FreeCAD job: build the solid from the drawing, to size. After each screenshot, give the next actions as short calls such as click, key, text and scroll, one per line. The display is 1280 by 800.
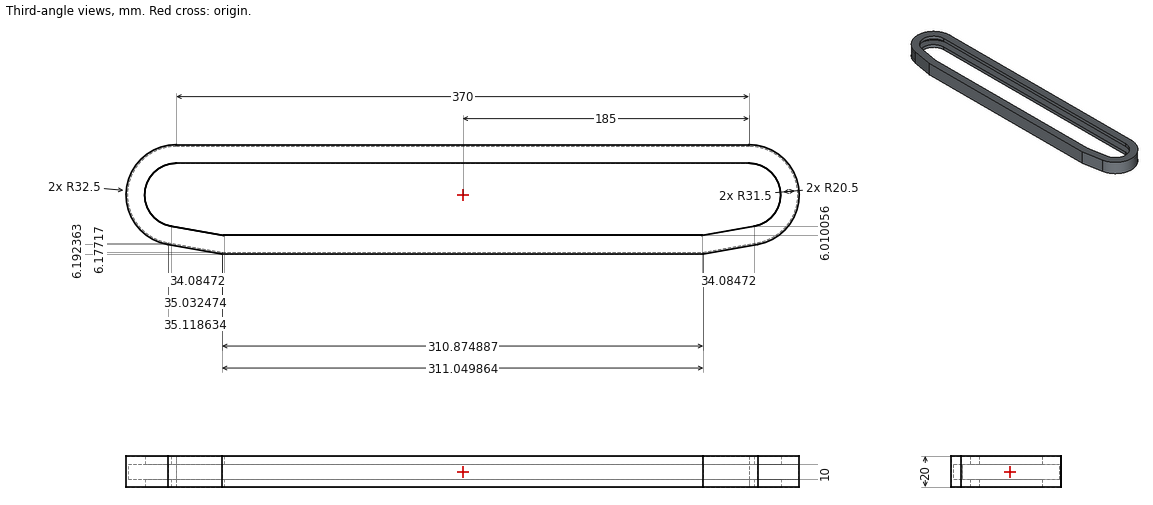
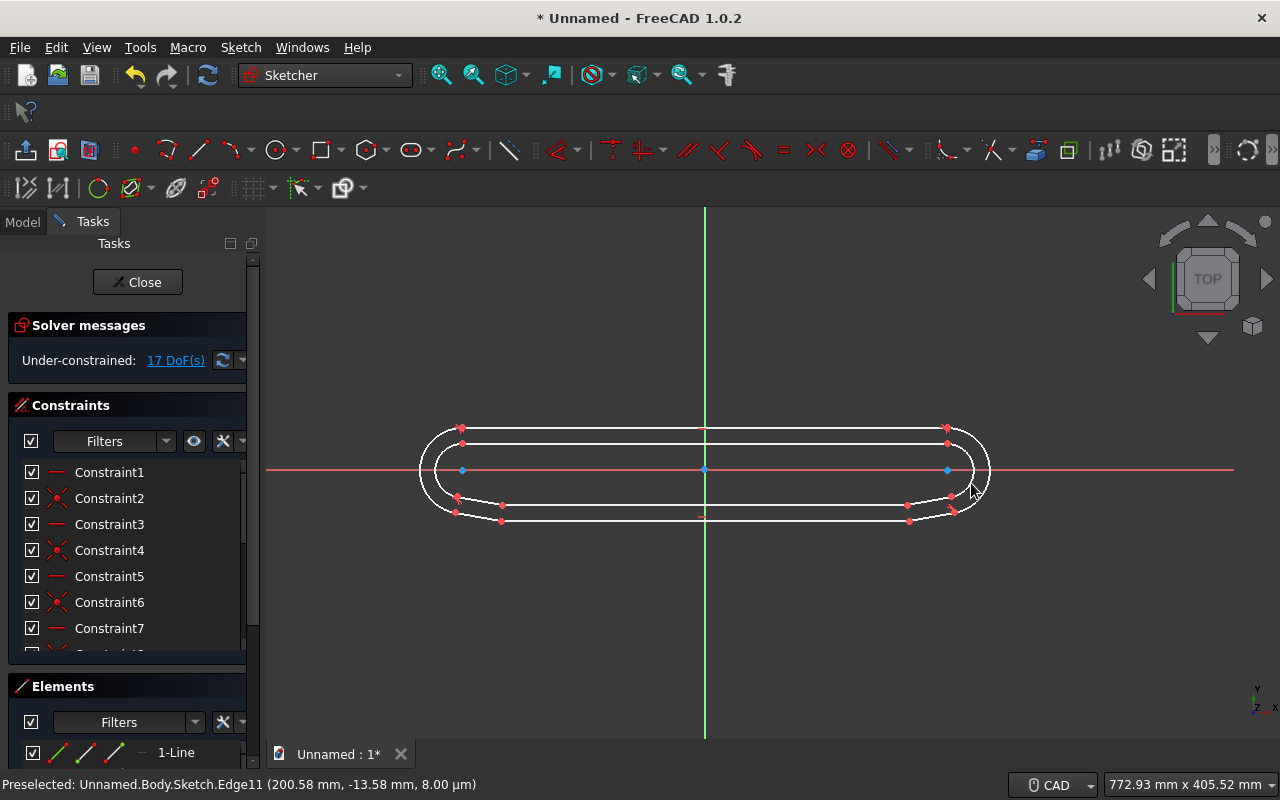
click(489, 503)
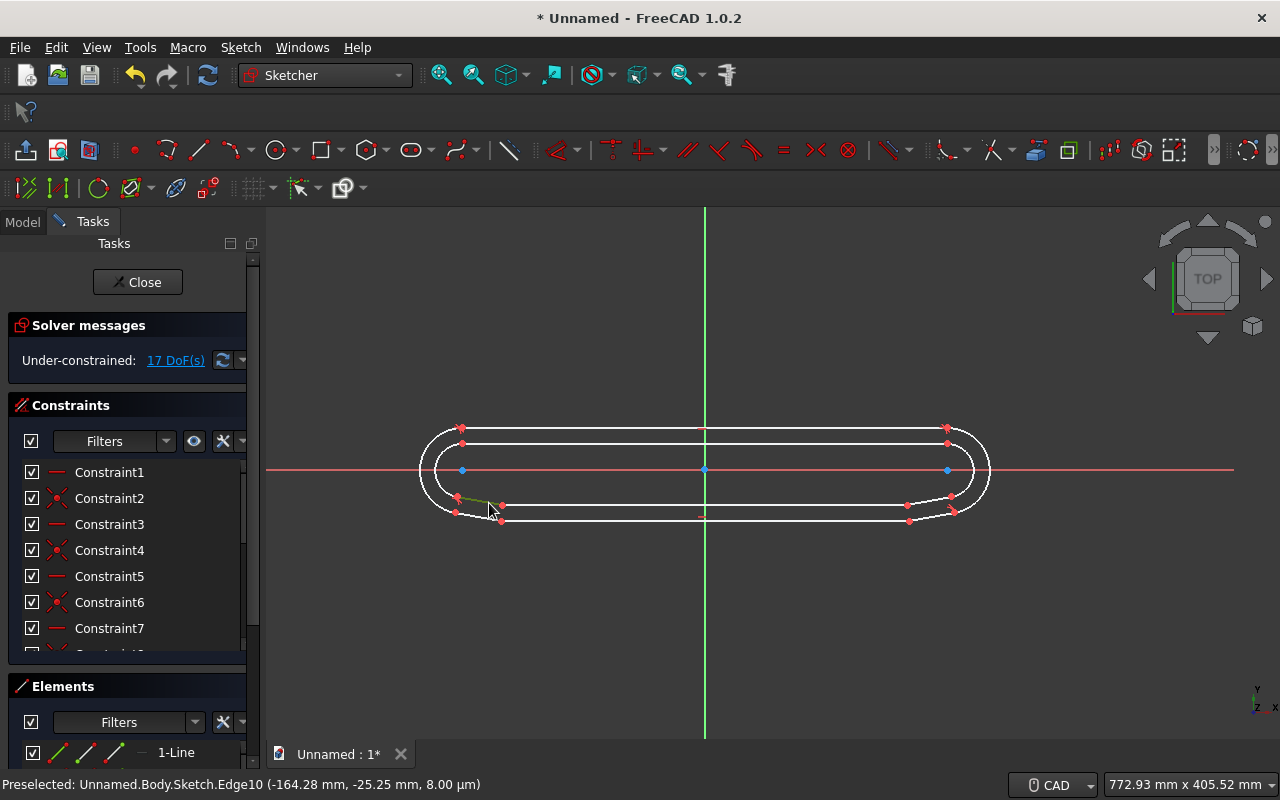
click(441, 454)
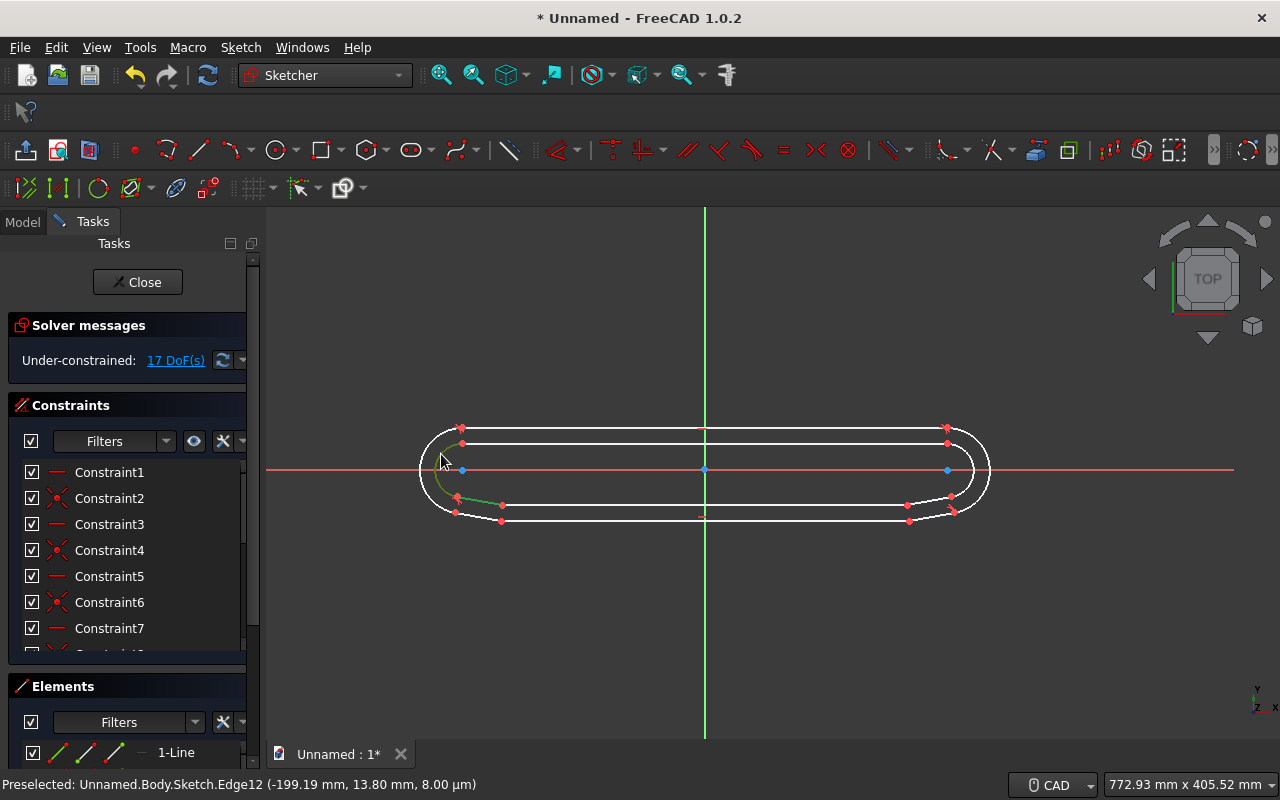
key(t)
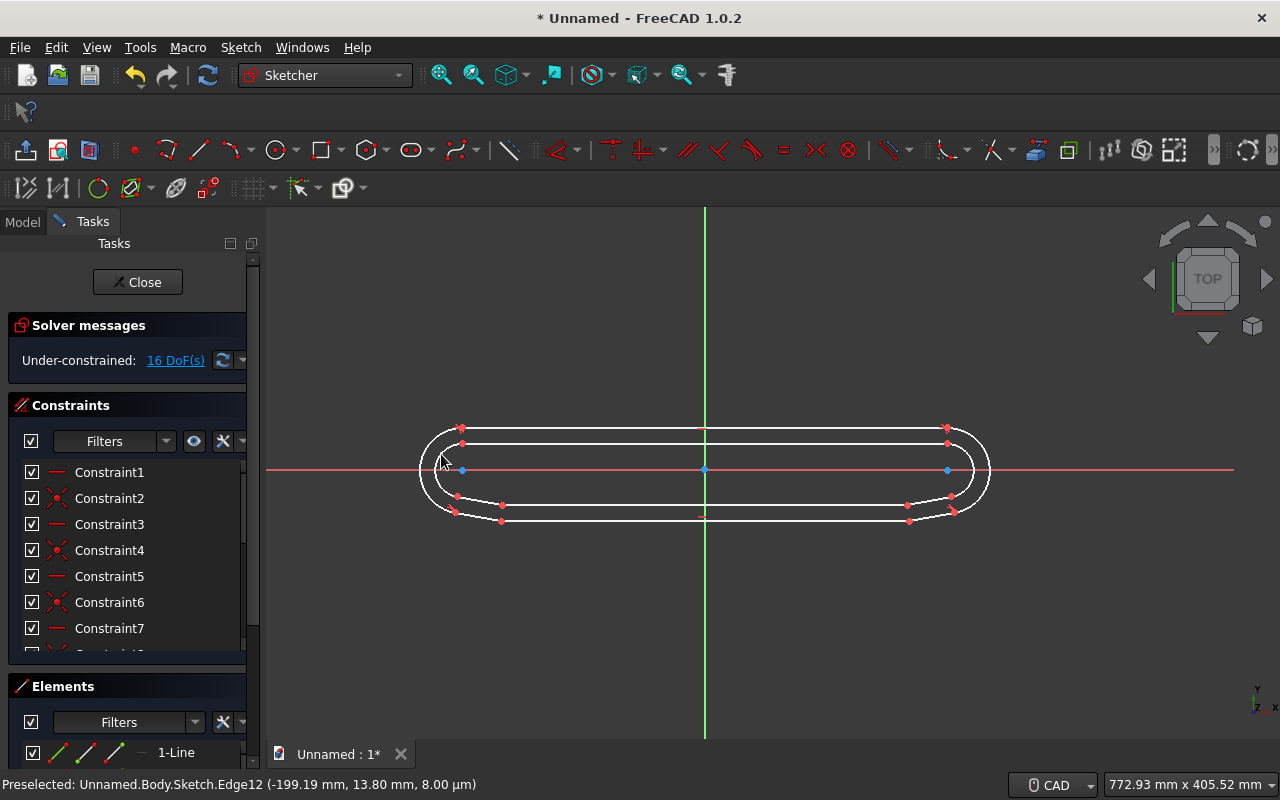
click(984, 492)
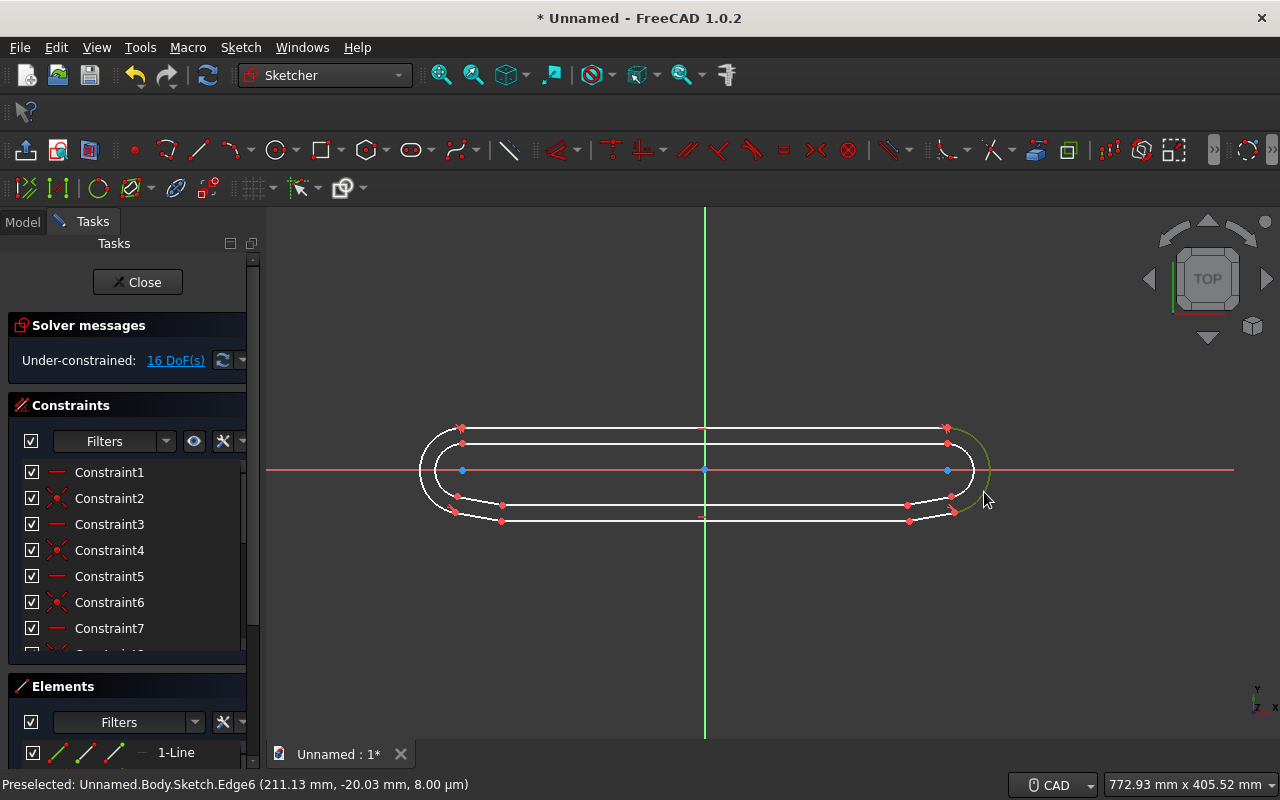
click(970, 484)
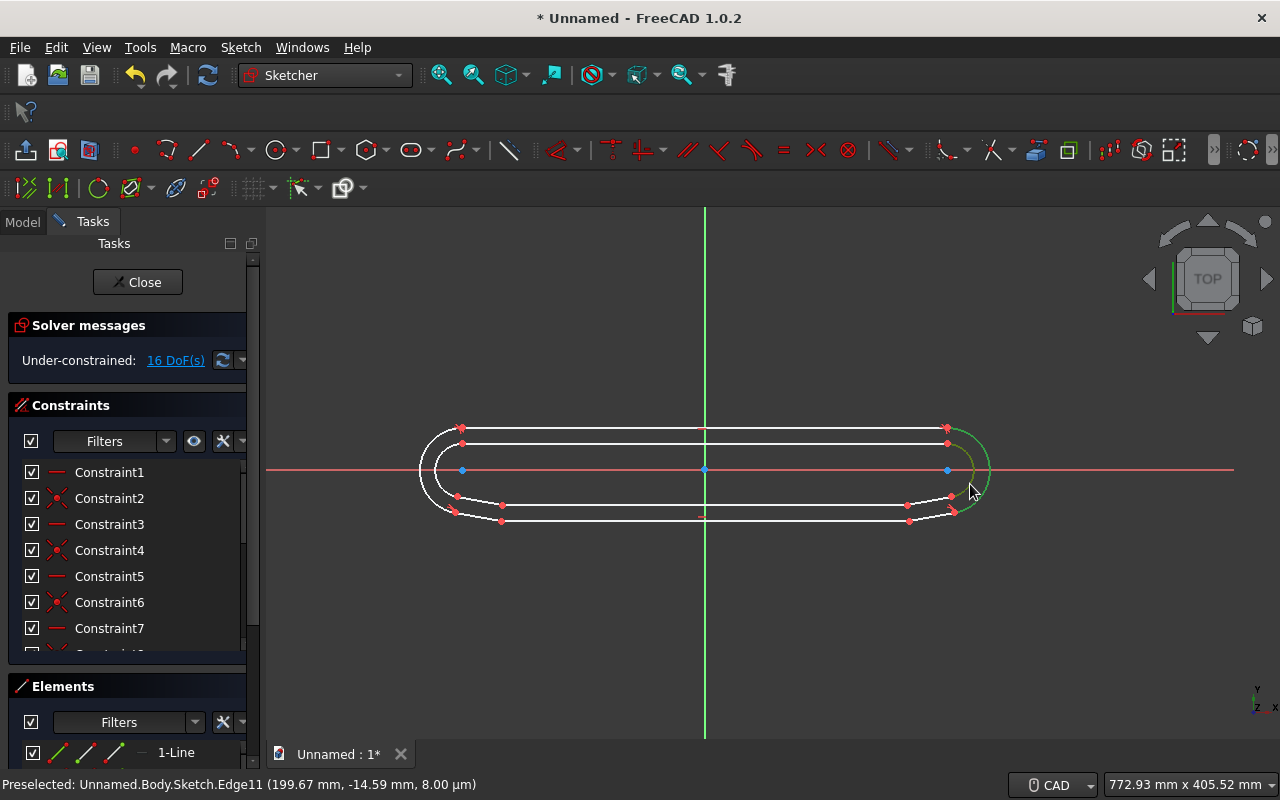
key(c)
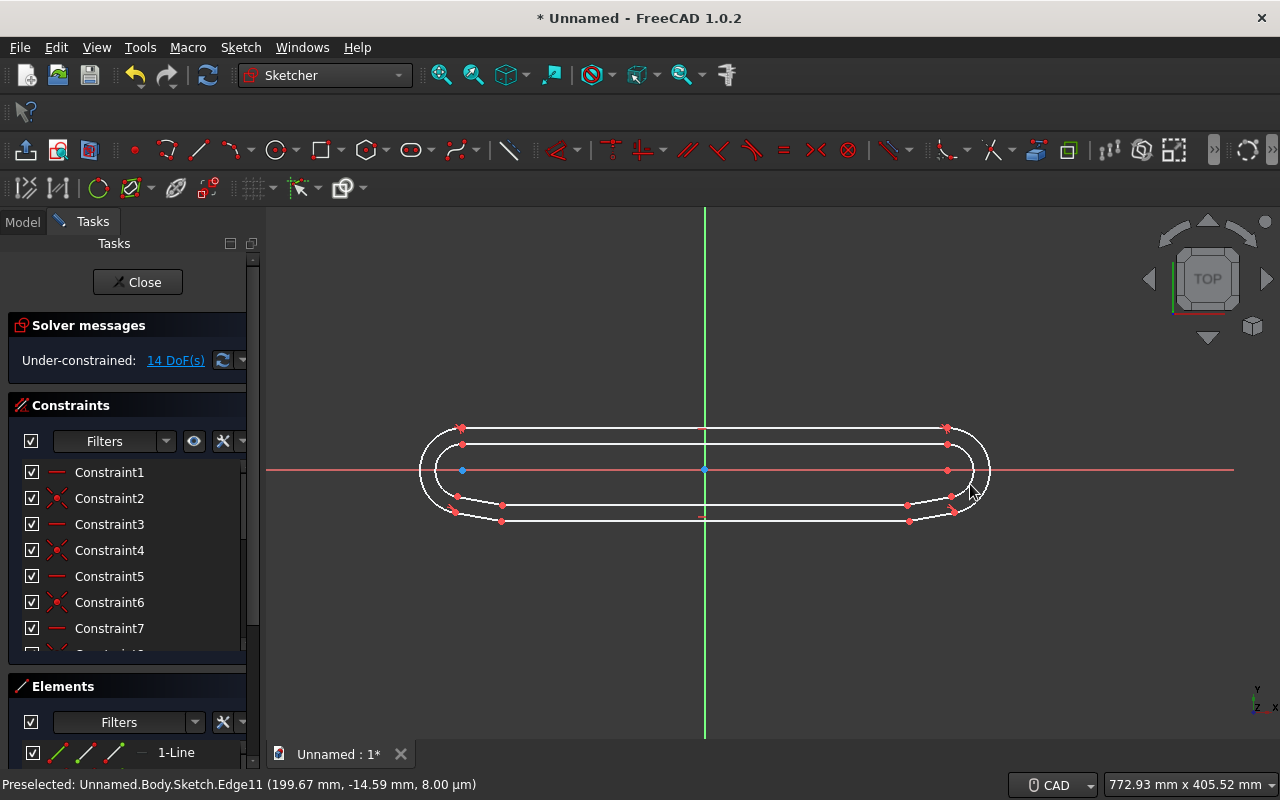
click(430, 444)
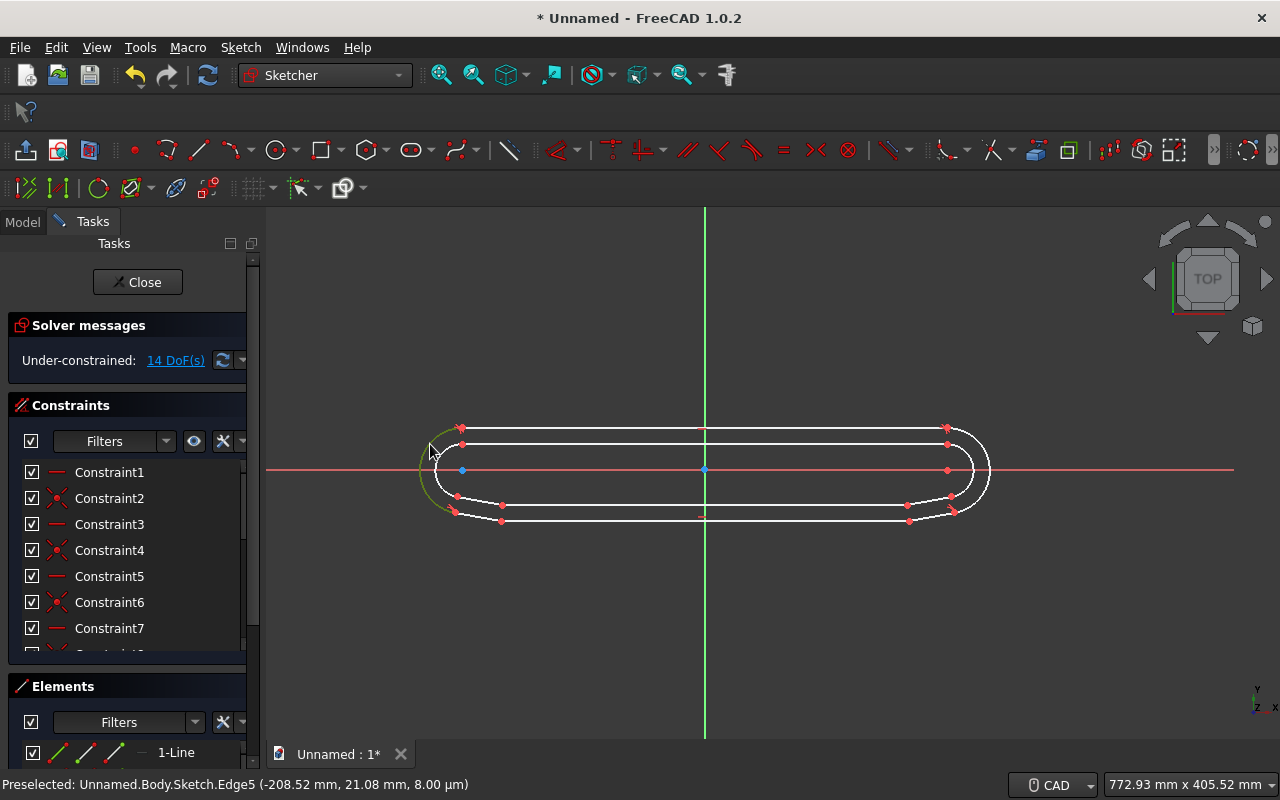
click(441, 454)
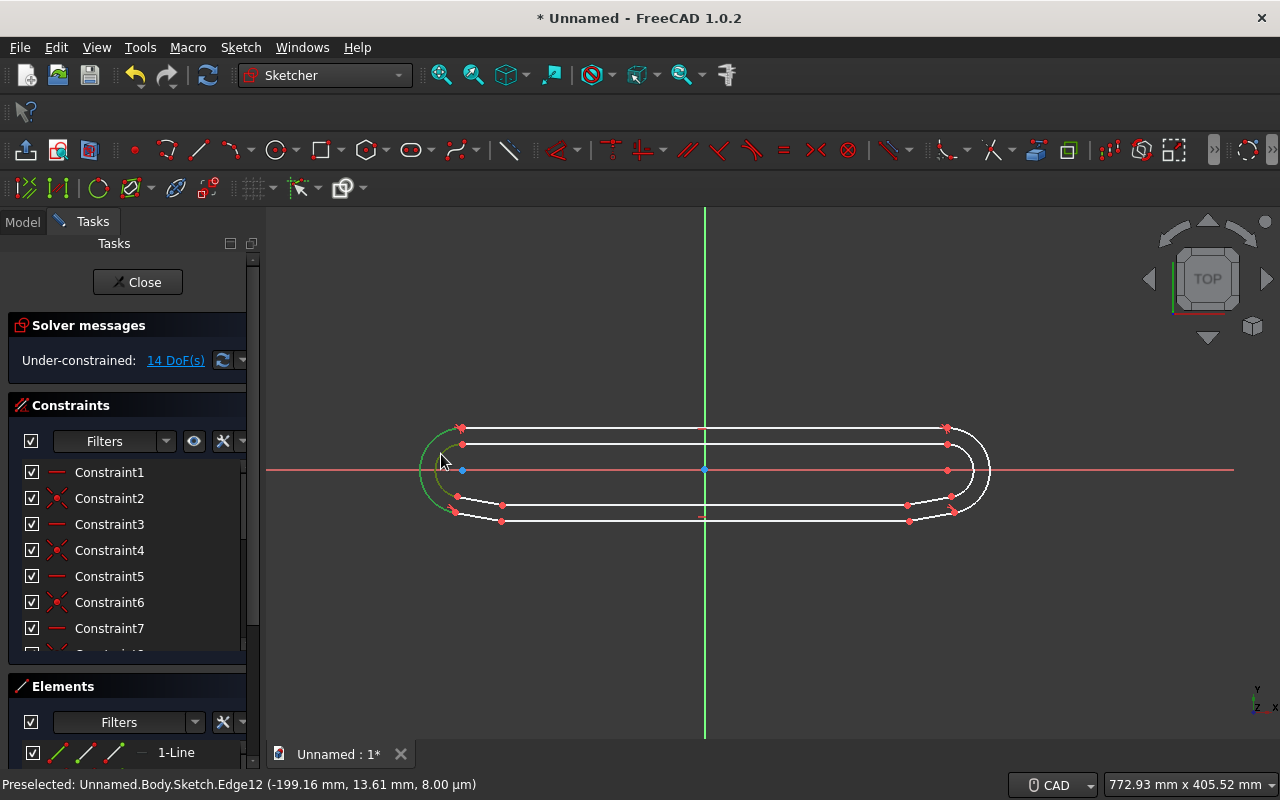
key(c)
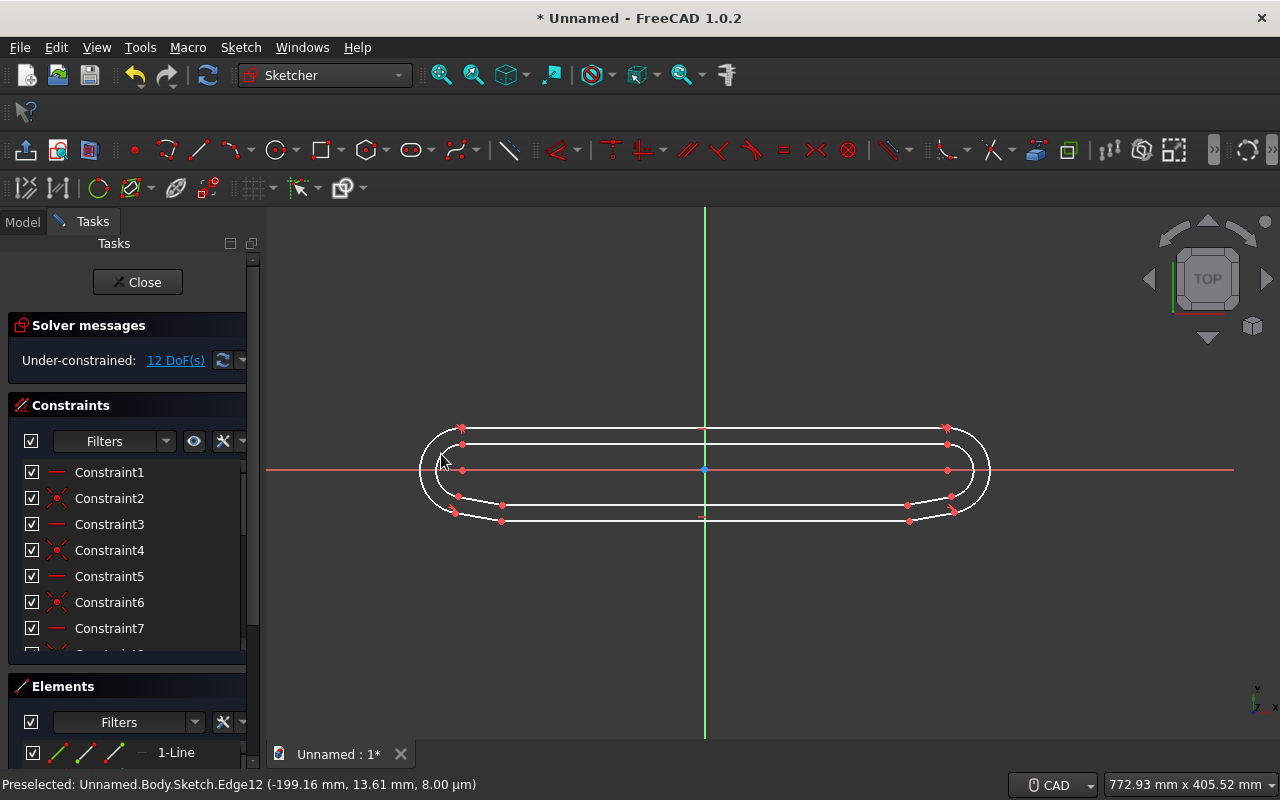
click(430, 444)